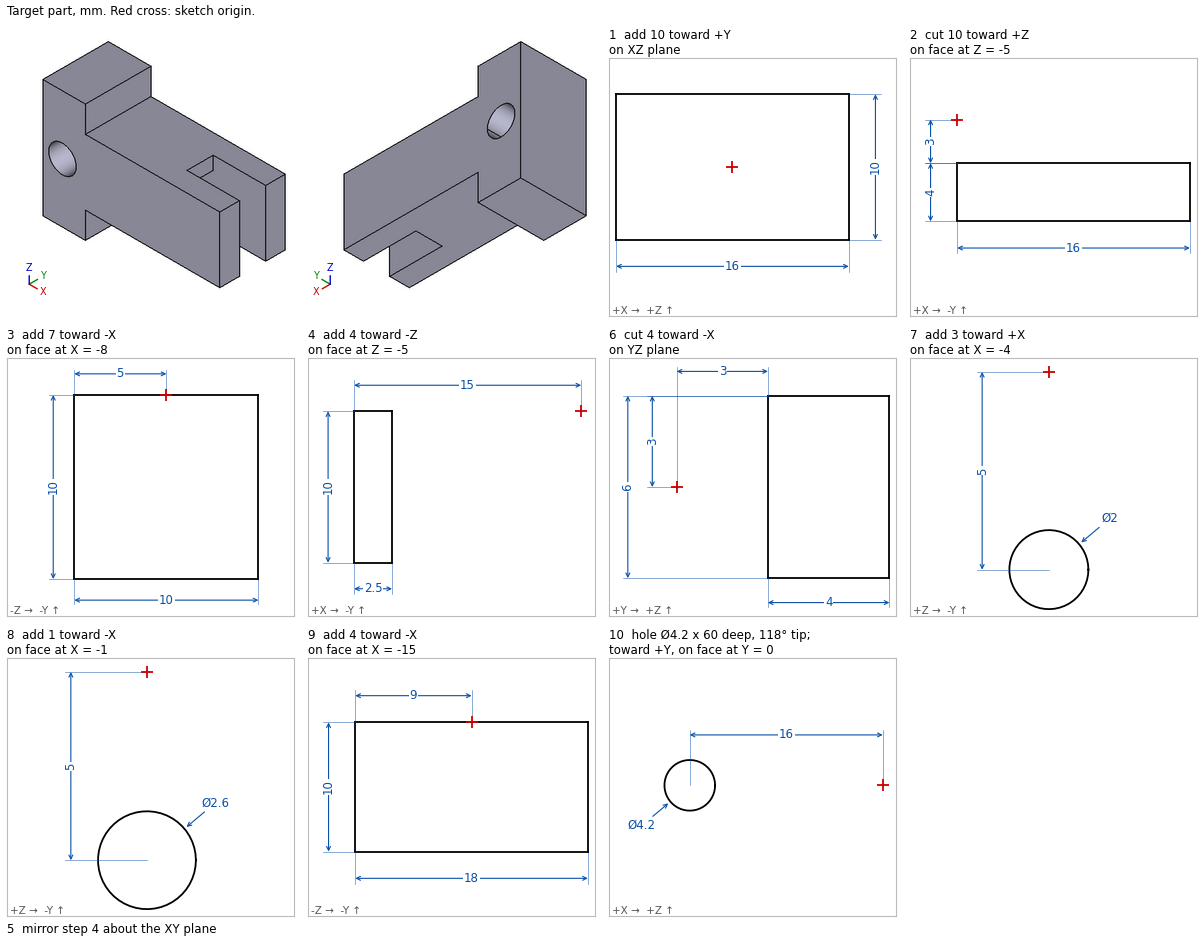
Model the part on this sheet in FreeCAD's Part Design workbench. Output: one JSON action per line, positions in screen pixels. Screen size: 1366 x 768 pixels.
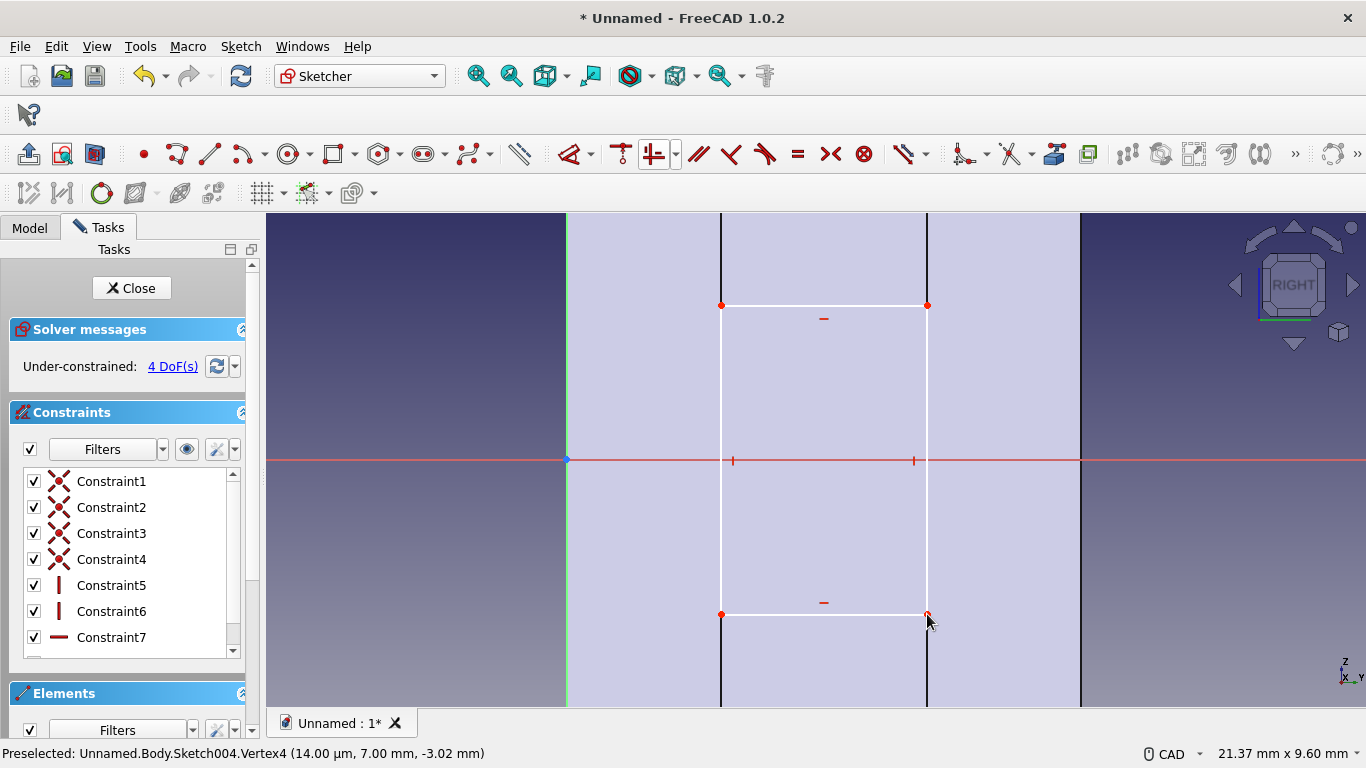
{"action": "left_click", "coordinate": [568, 154]}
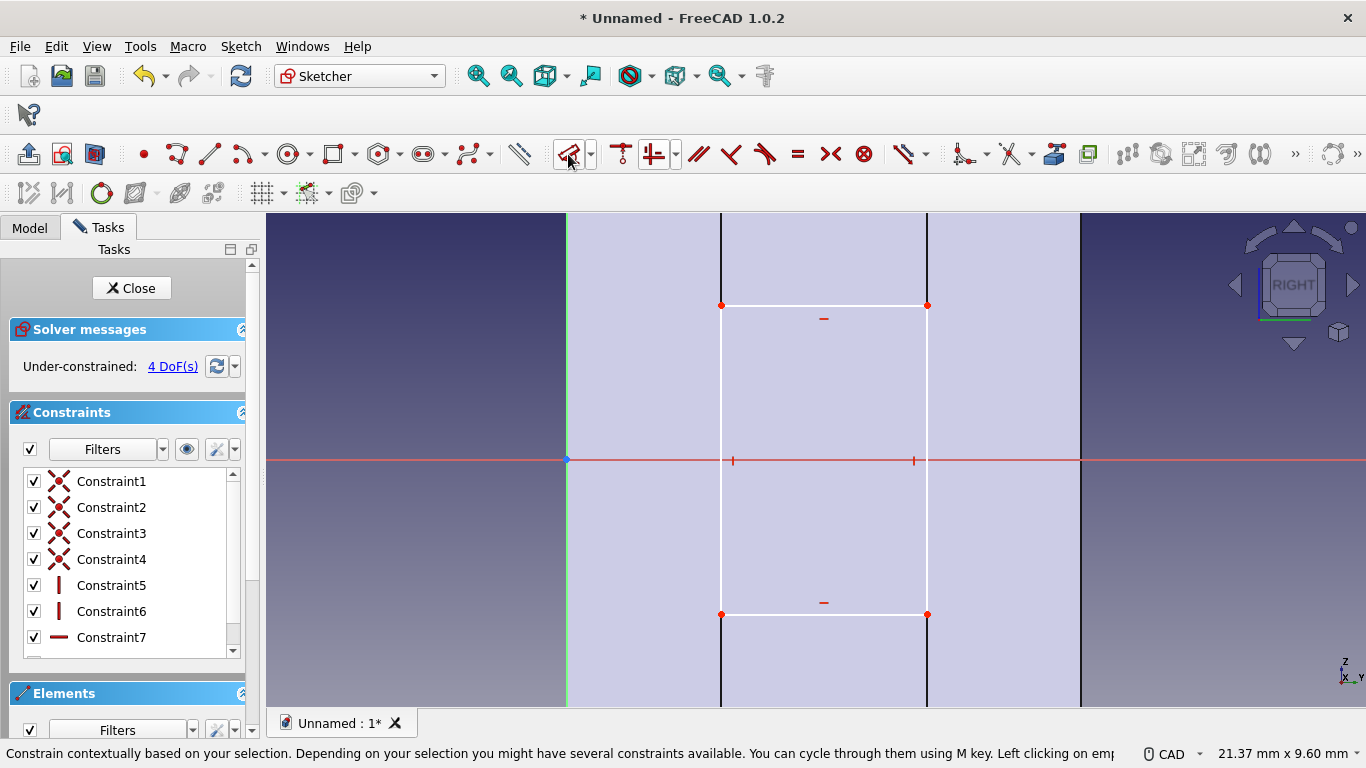
{"action": "left_click", "coordinate": [721, 399]}
{"action": "left_click", "coordinate": [687, 389]}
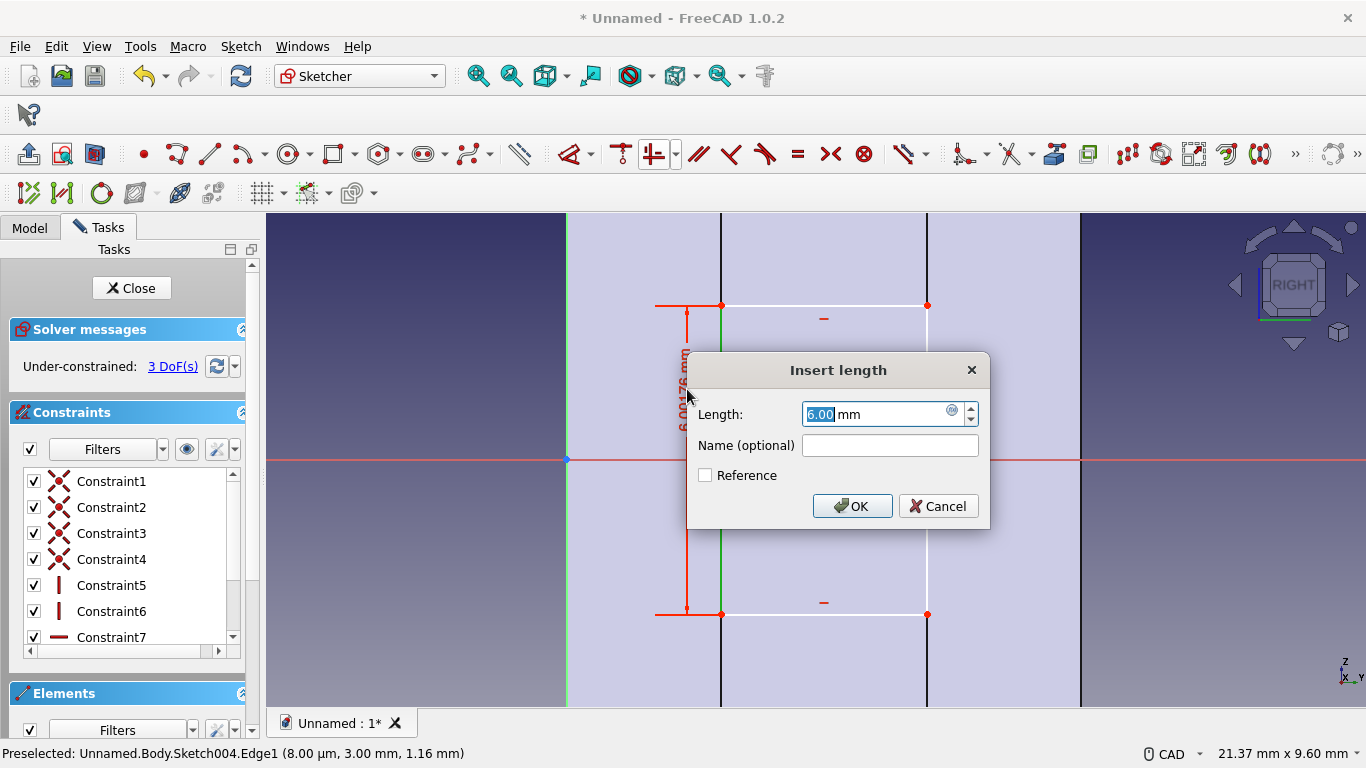
{"action": "type", "text": "6"}
{"action": "key", "text": "Return"}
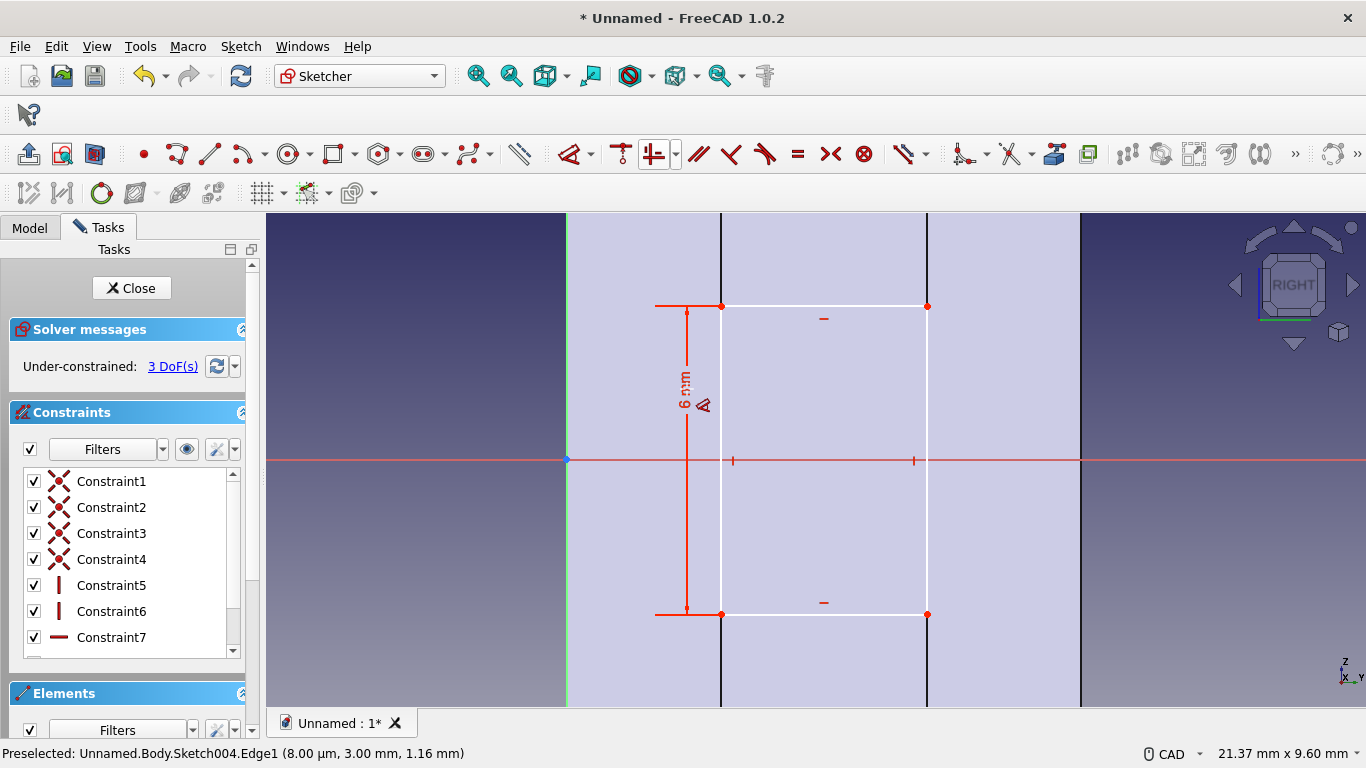
{"action": "left_click", "coordinate": [783, 615]}
{"action": "left_click", "coordinate": [824, 649]}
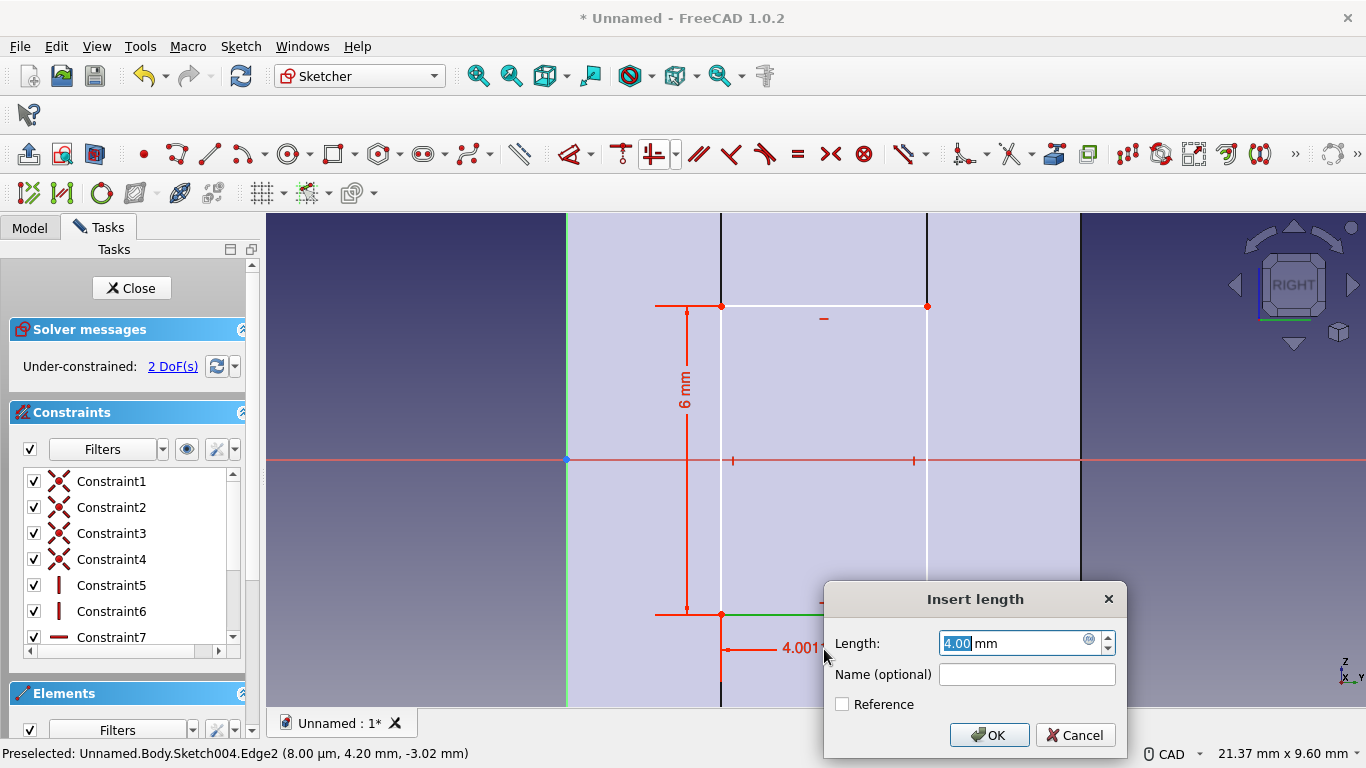
{"action": "type", "text": "4"}
{"action": "key", "text": "Return"}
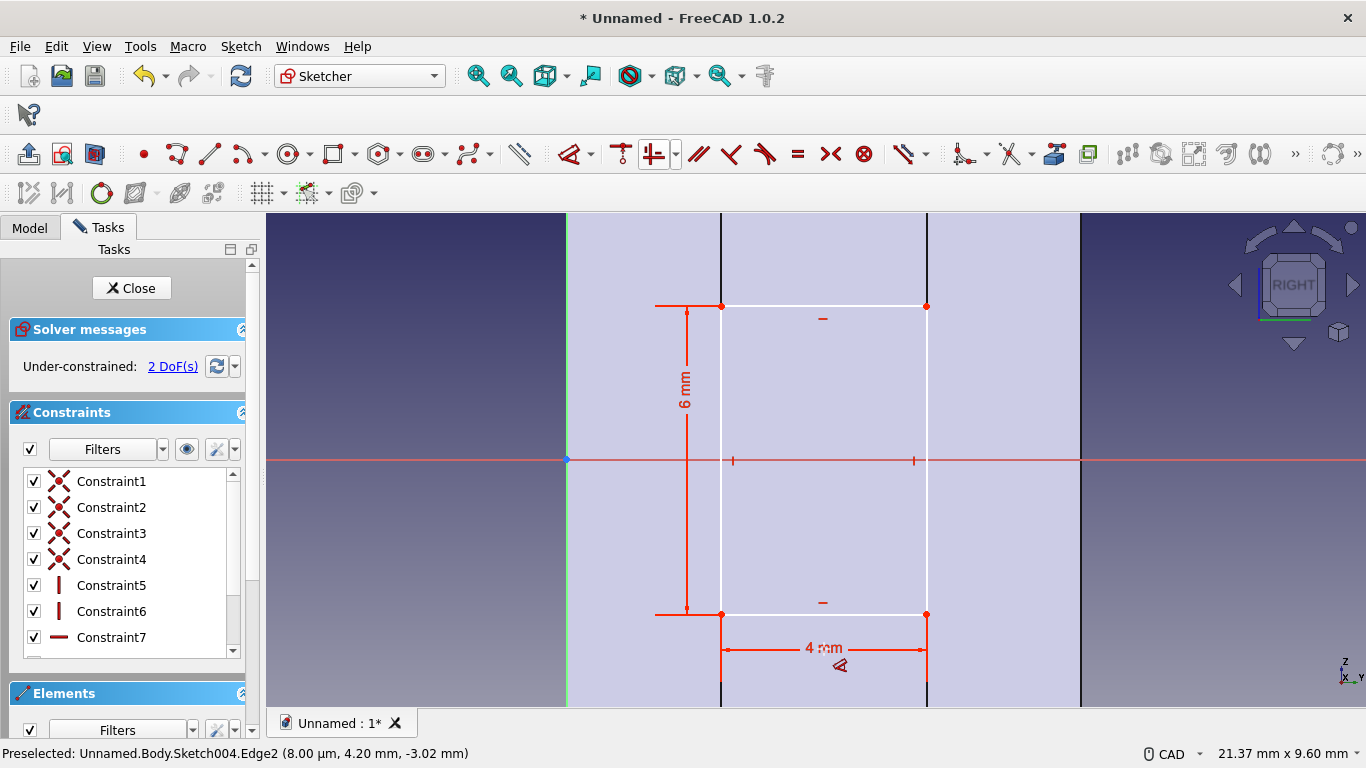
{"action": "left_click", "coordinate": [721, 306]}
{"action": "left_click", "coordinate": [644, 272]}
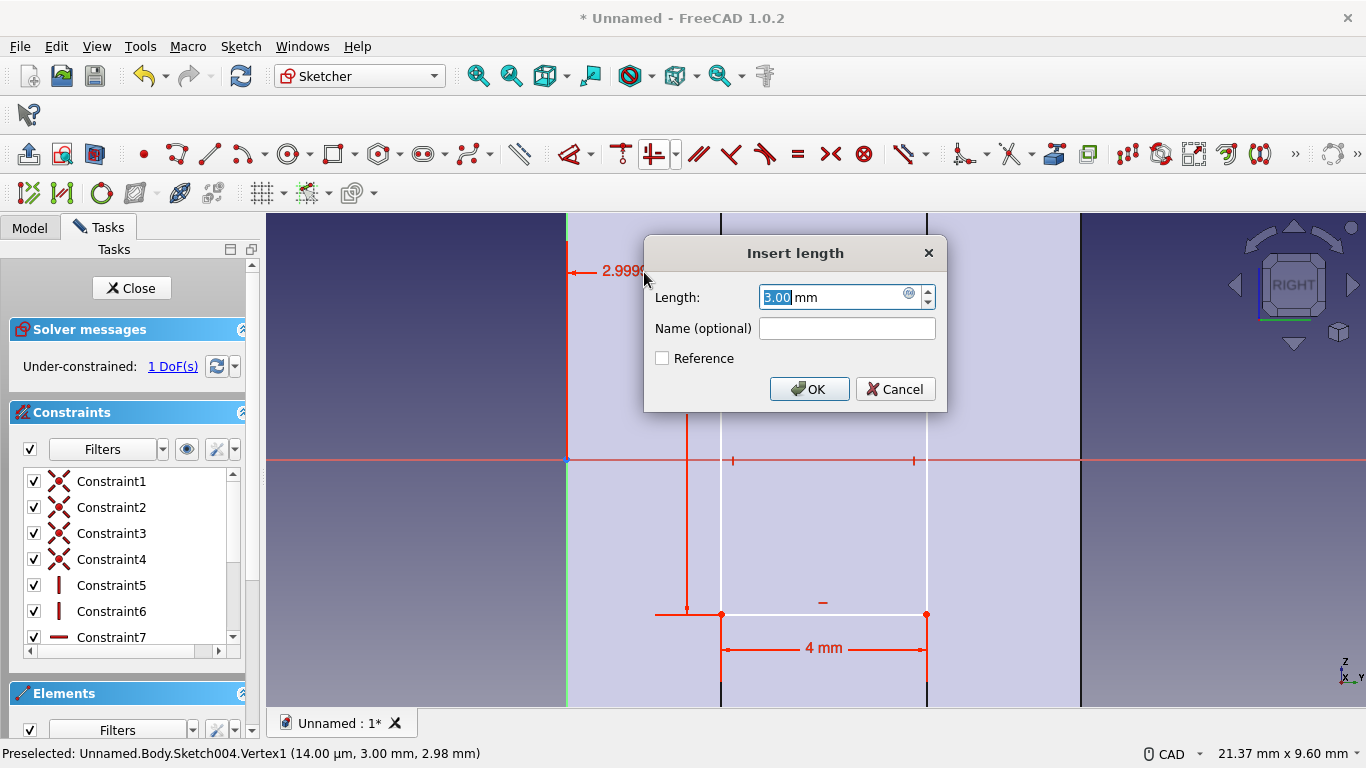
{"action": "type", "text": "3"}
{"action": "key", "text": "Return"}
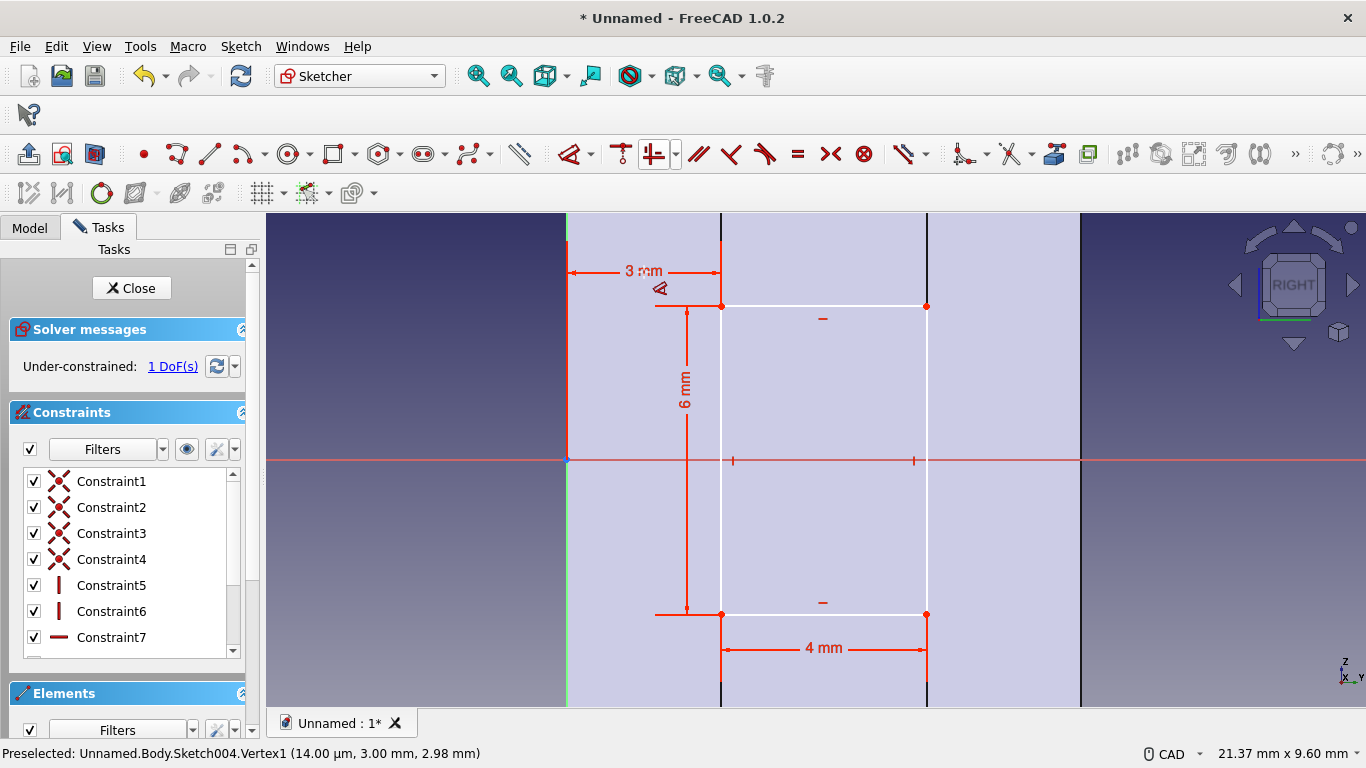
{"action": "left_click", "coordinate": [721, 306]}
{"action": "left_click", "coordinate": [533, 383]}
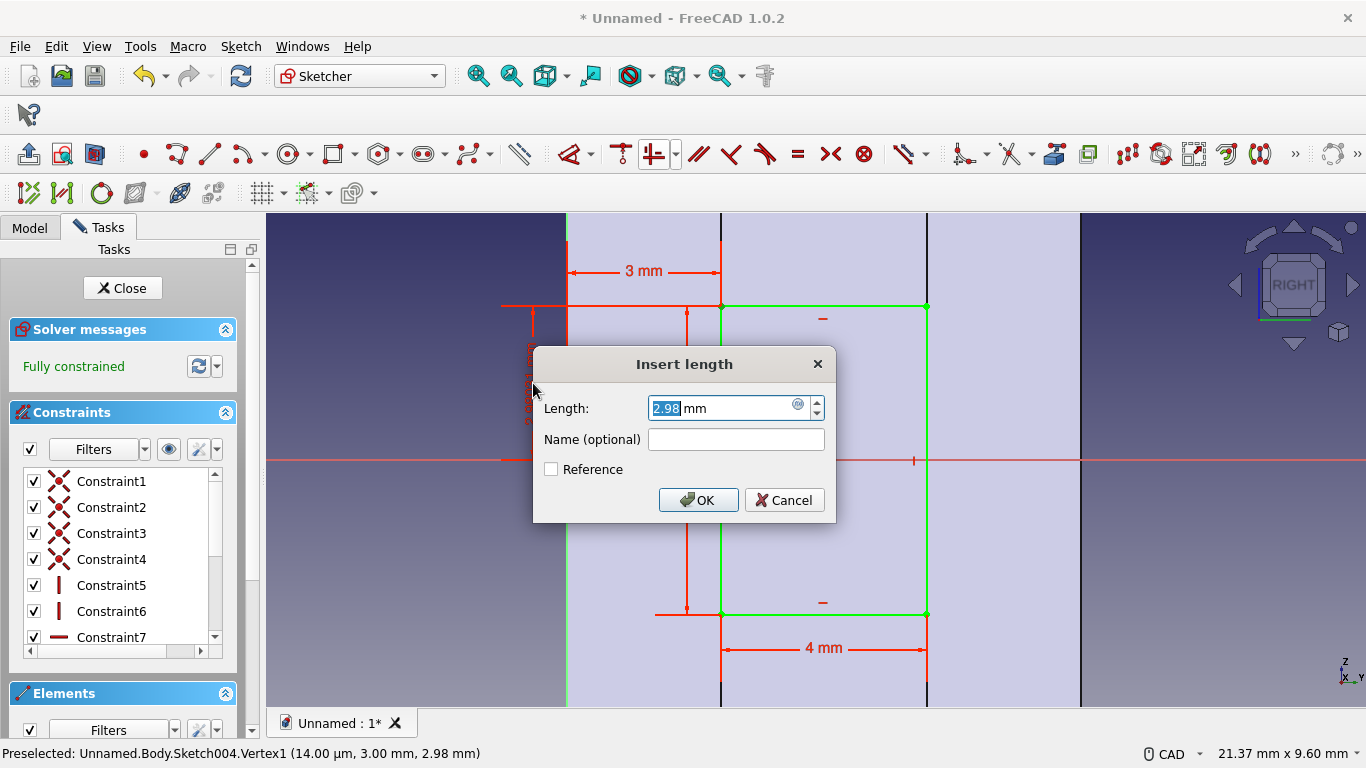
{"action": "type", "text": "3"}
{"action": "key", "text": "Return"}
{"action": "key", "text": "Escape"}